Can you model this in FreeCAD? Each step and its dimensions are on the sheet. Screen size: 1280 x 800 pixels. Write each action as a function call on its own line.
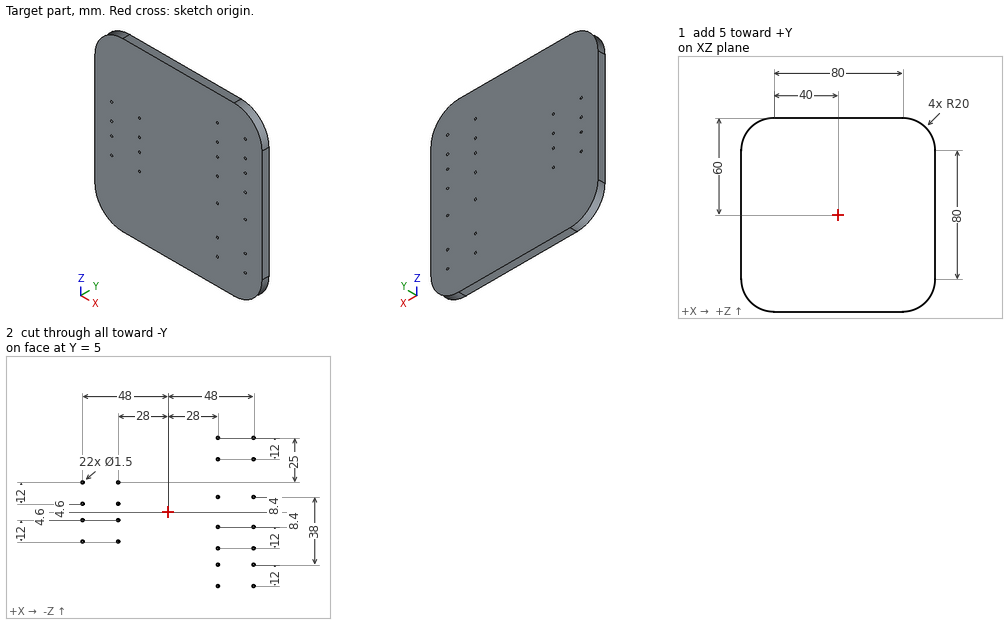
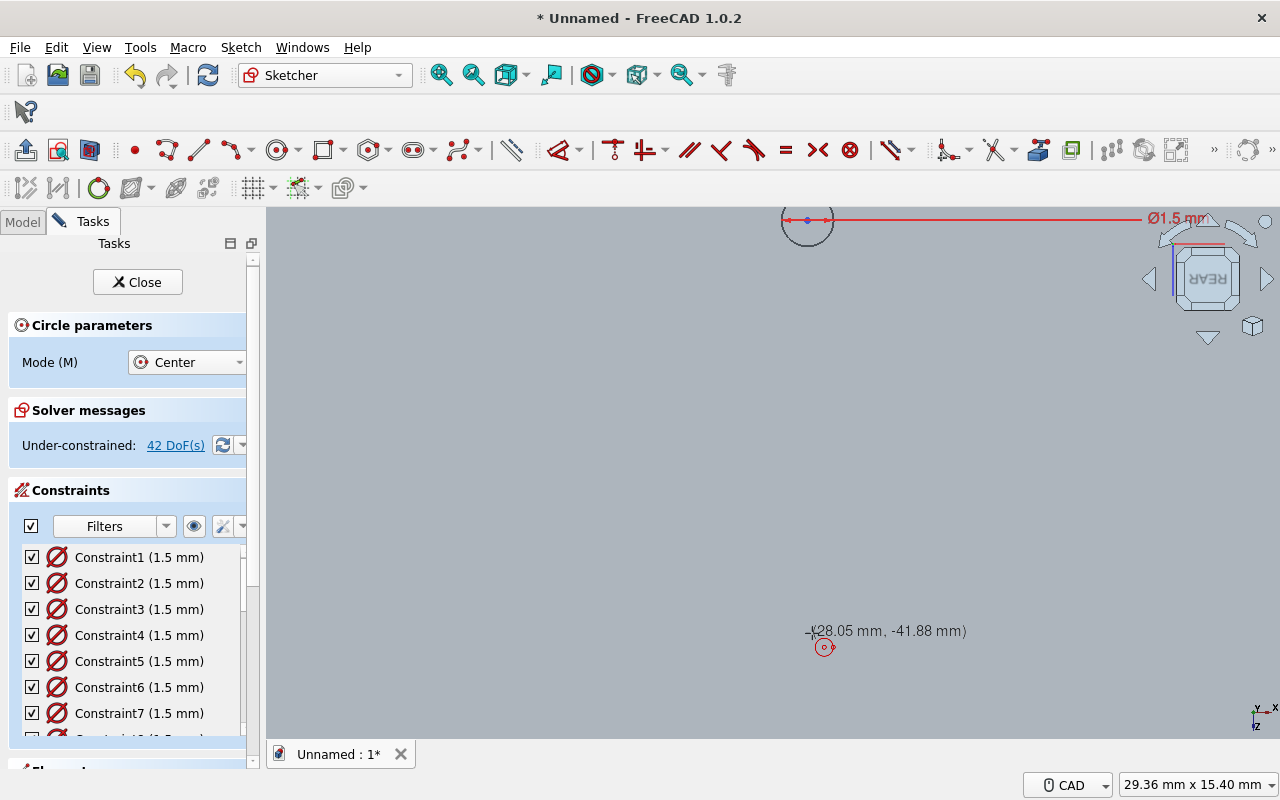
scroll(812, 633, down, 11)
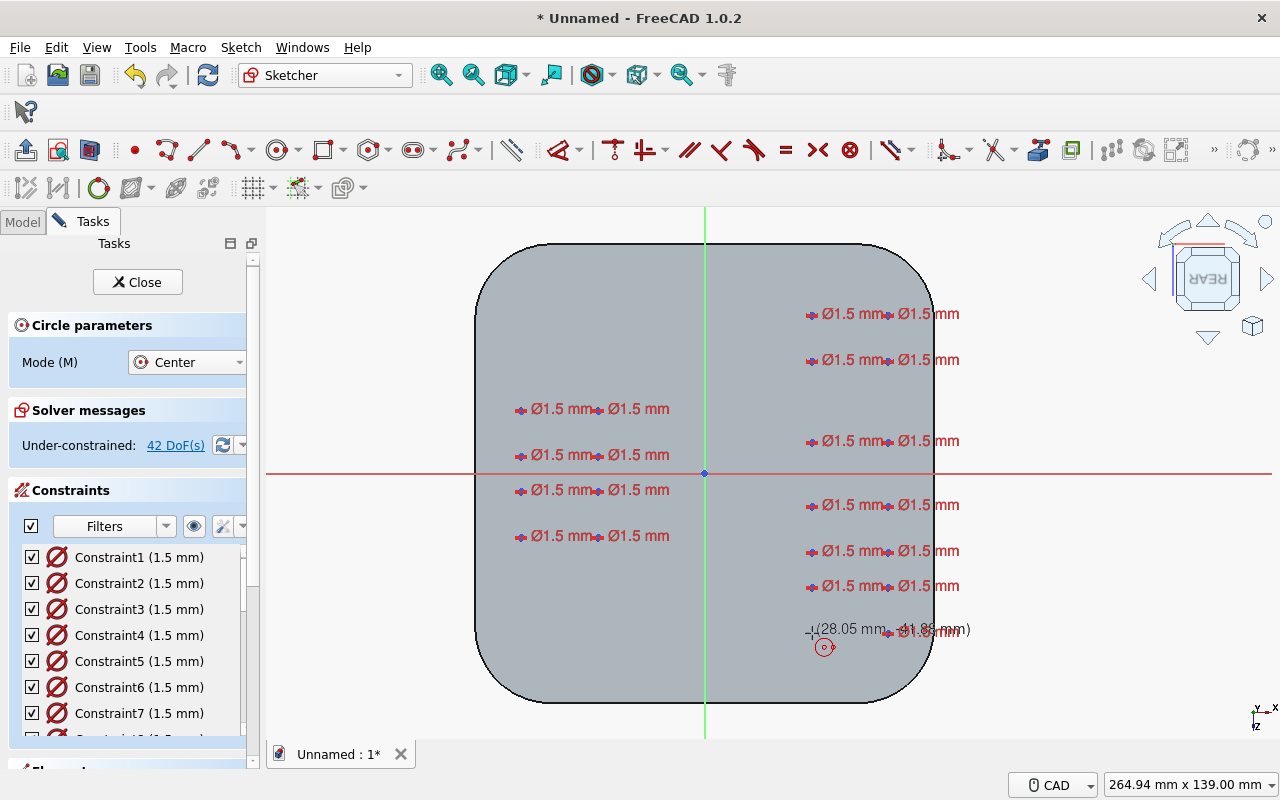
click(812, 633)
move(814, 631)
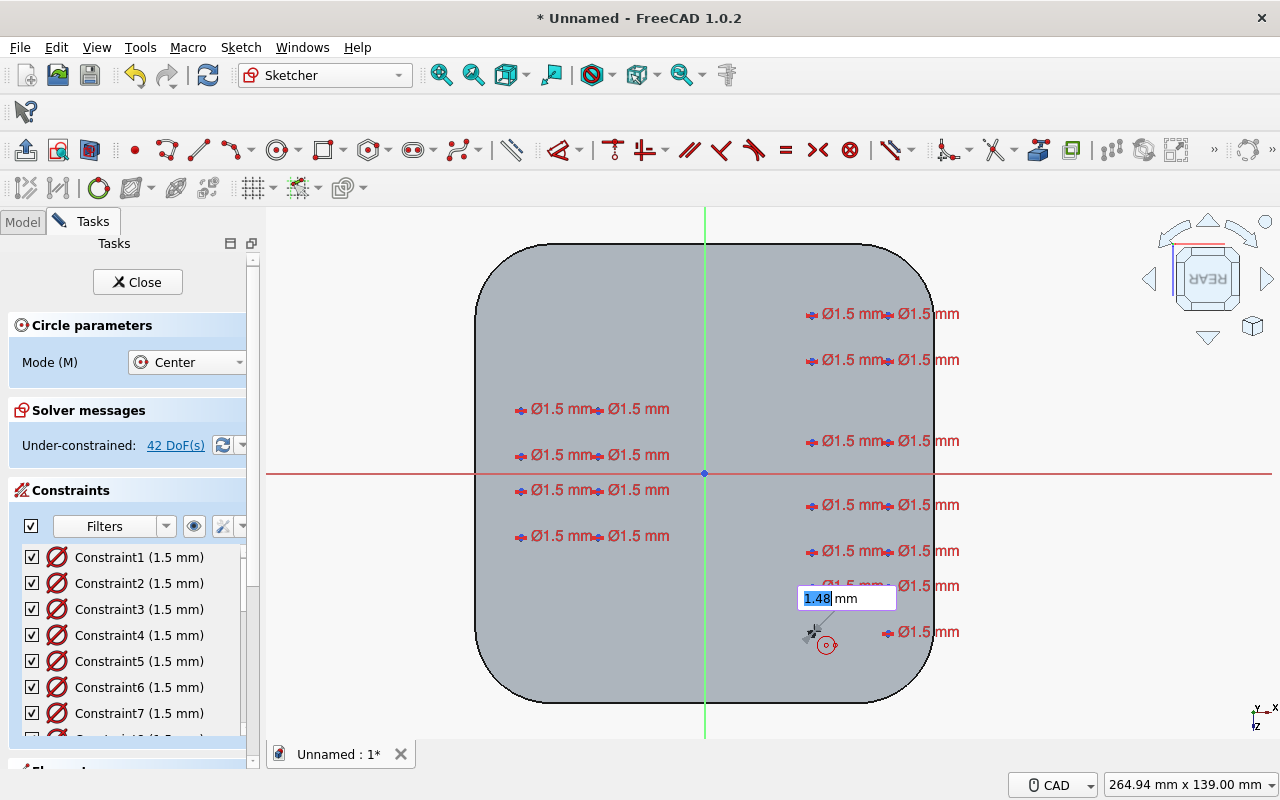
text(1.5)
key(Return)
key(Escape)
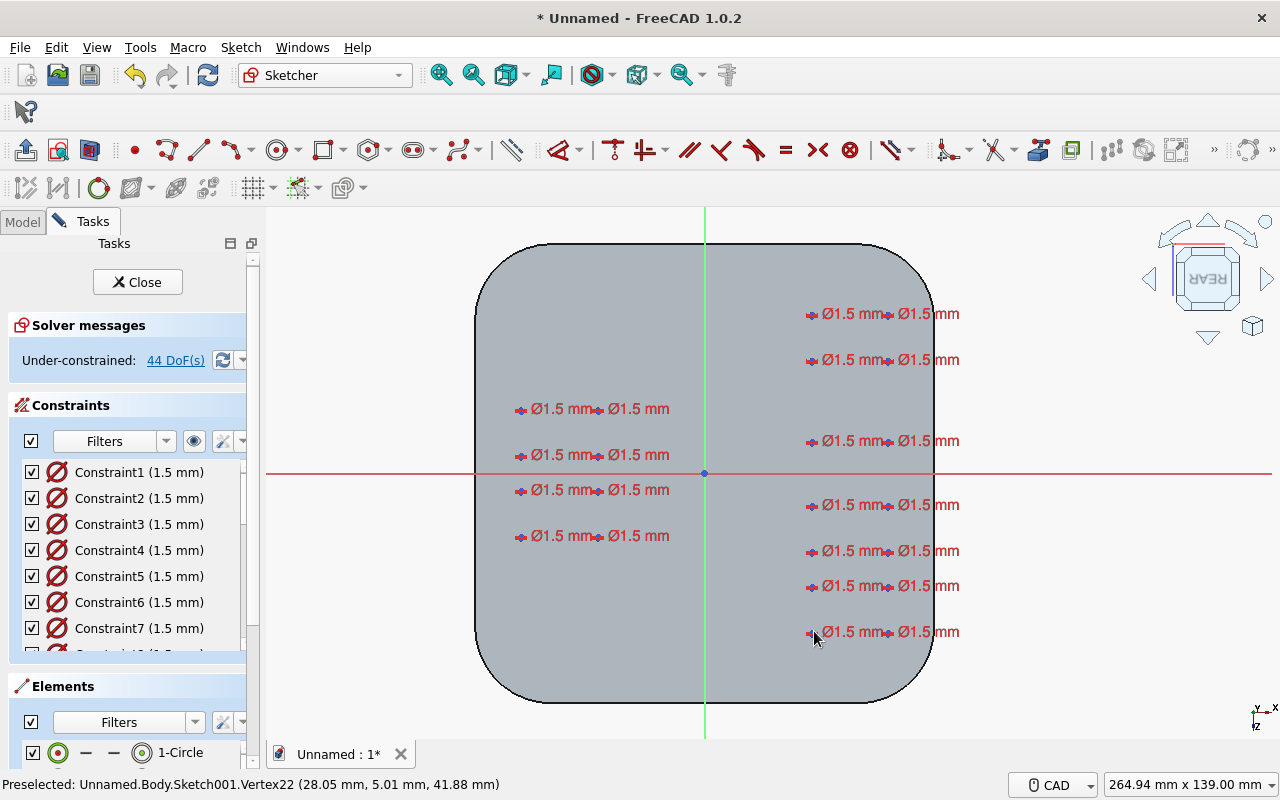
click(521, 411)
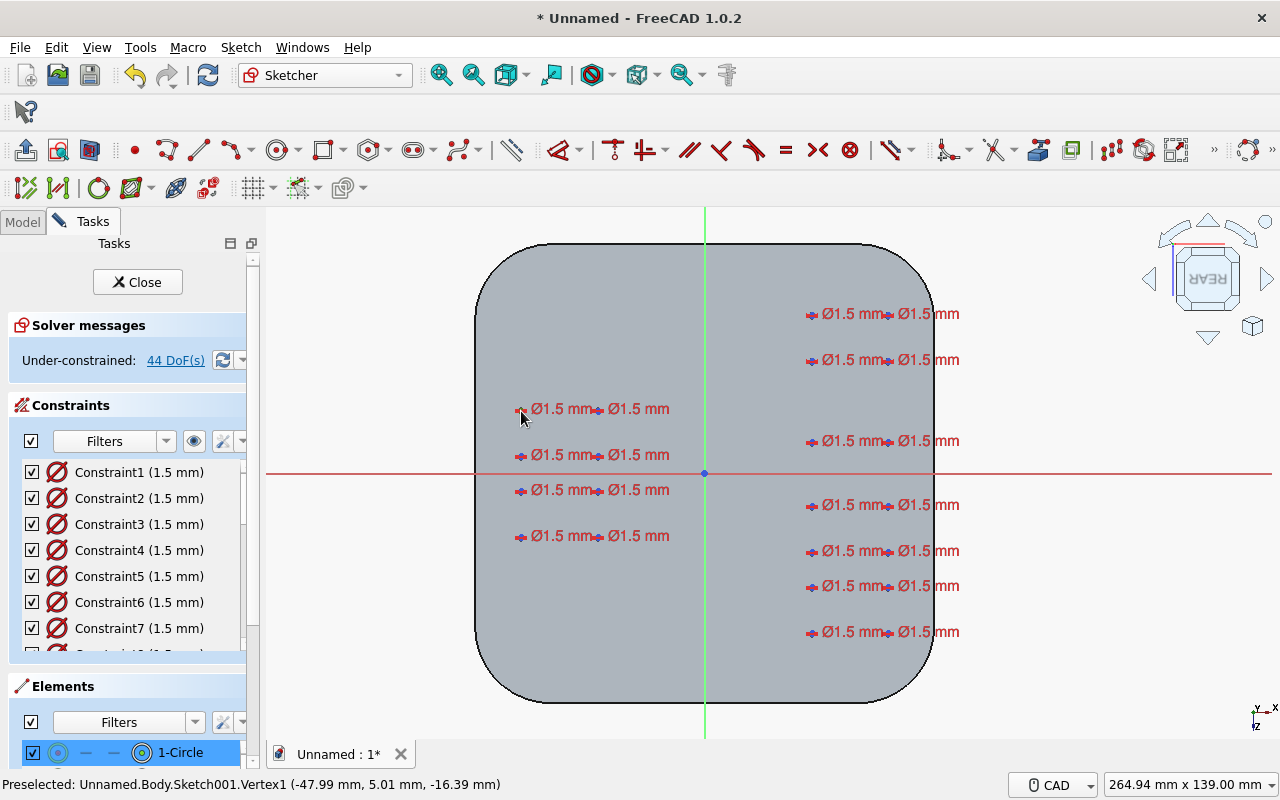
click(598, 411)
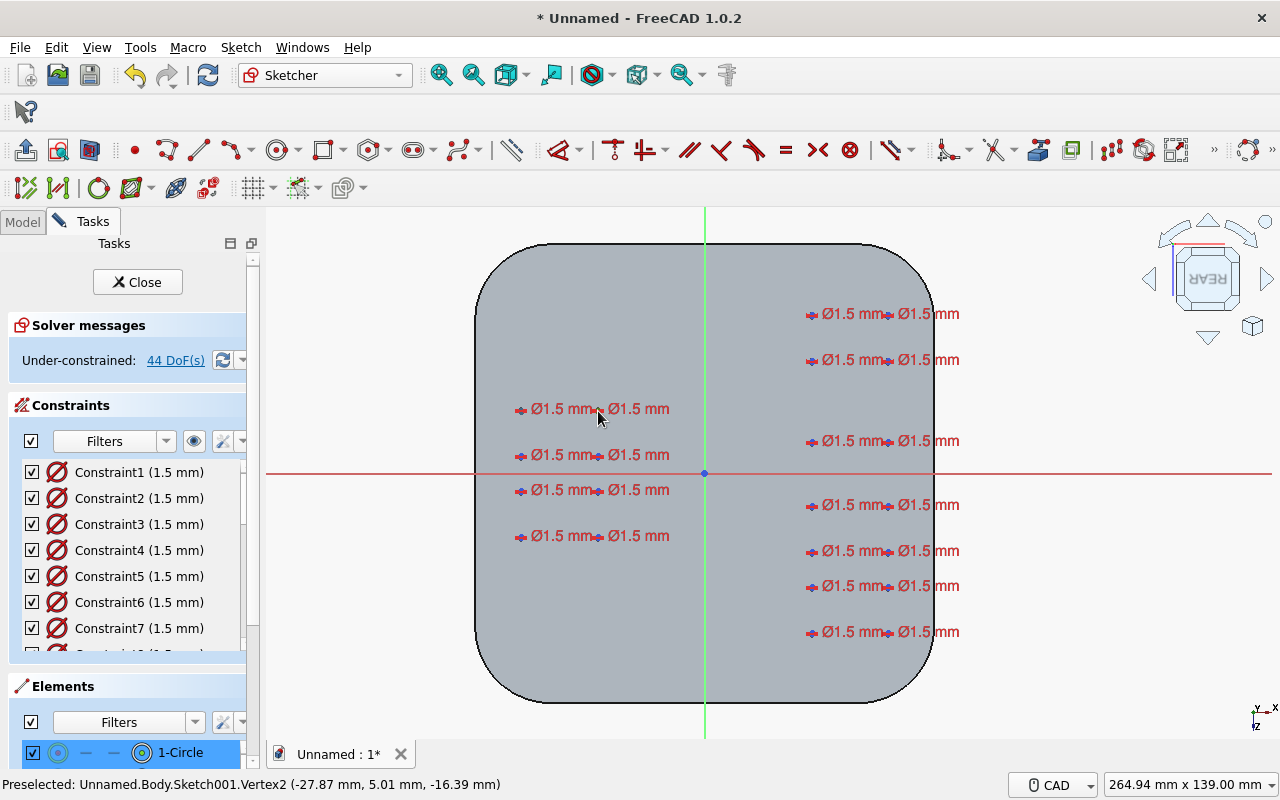
click(668, 150)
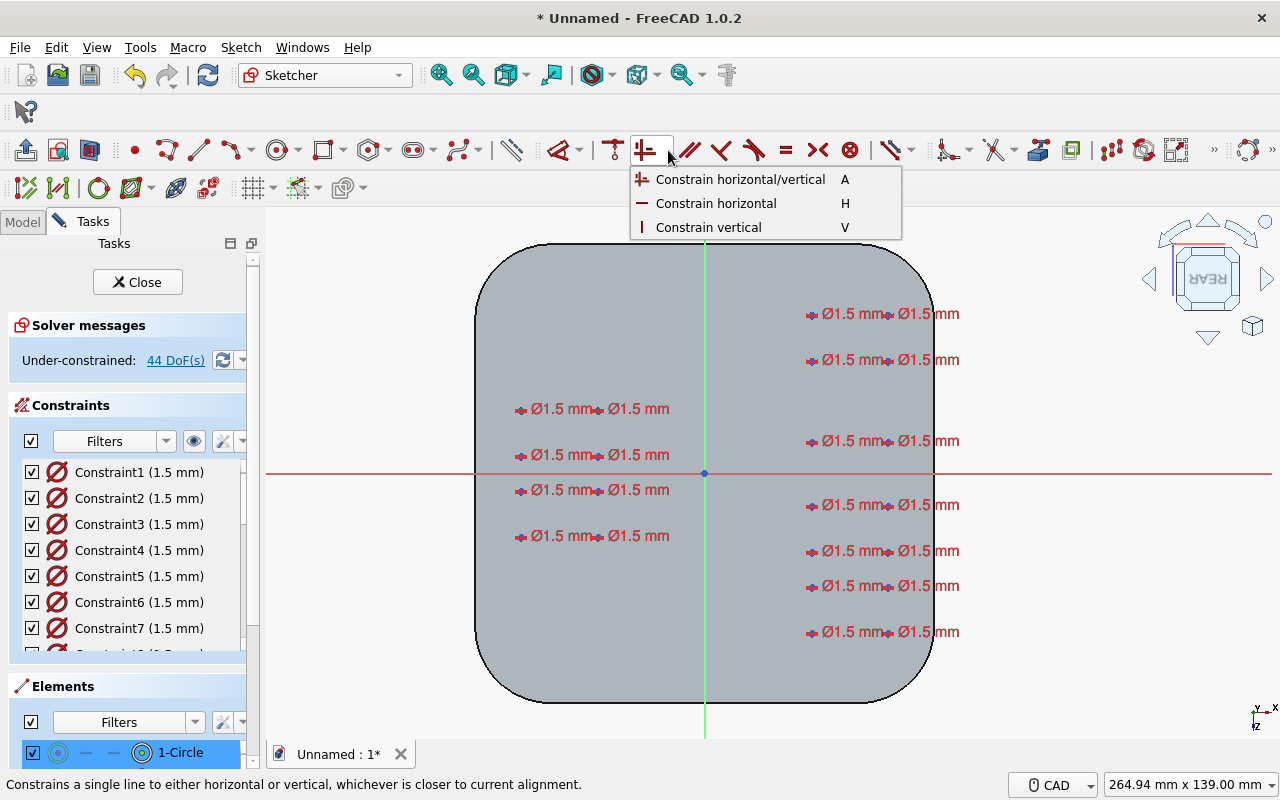
click(766, 203)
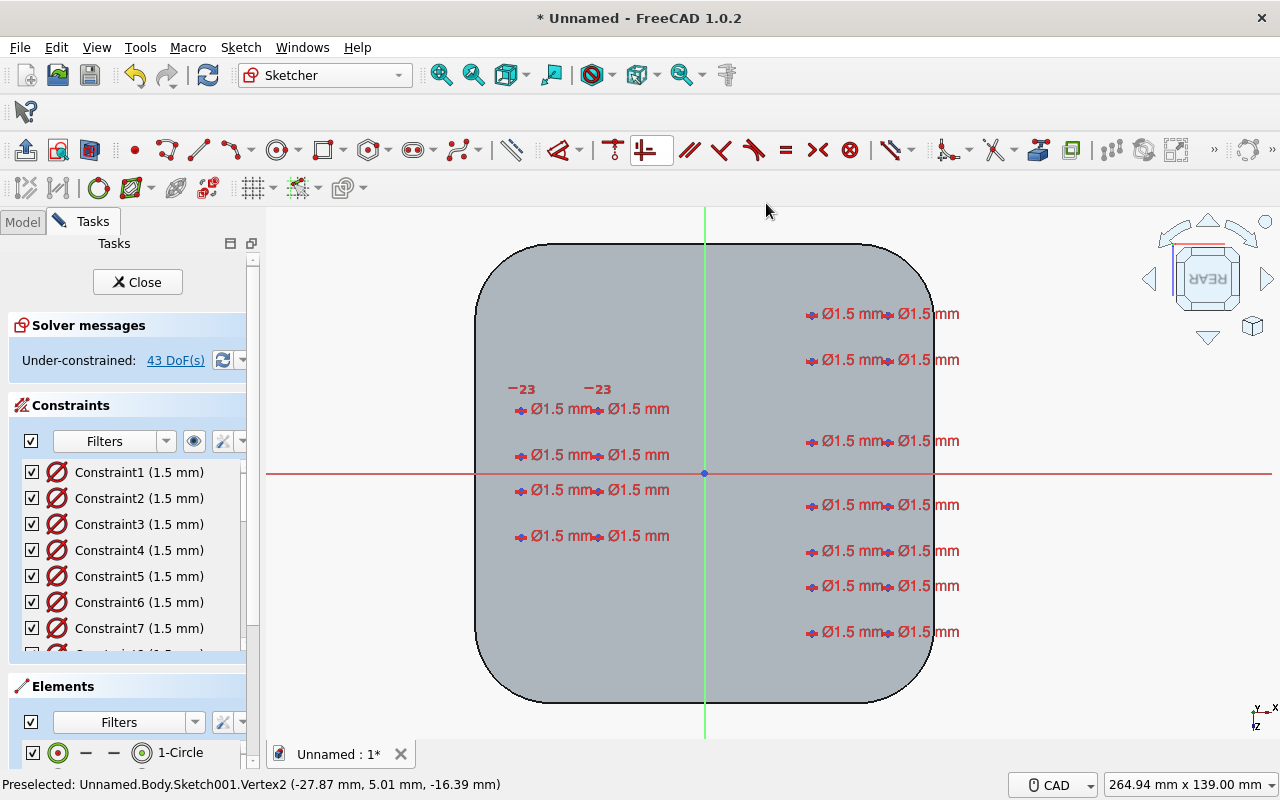
click(521, 411)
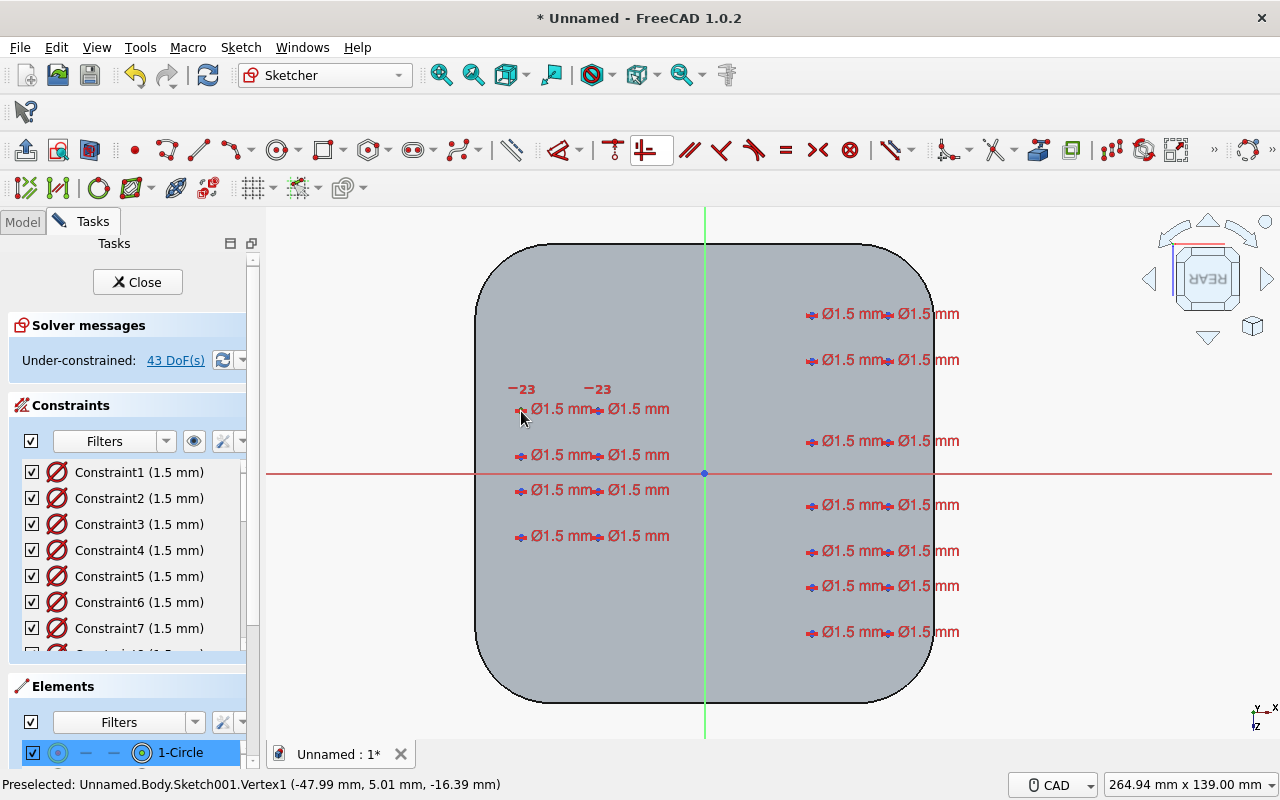
click(521, 457)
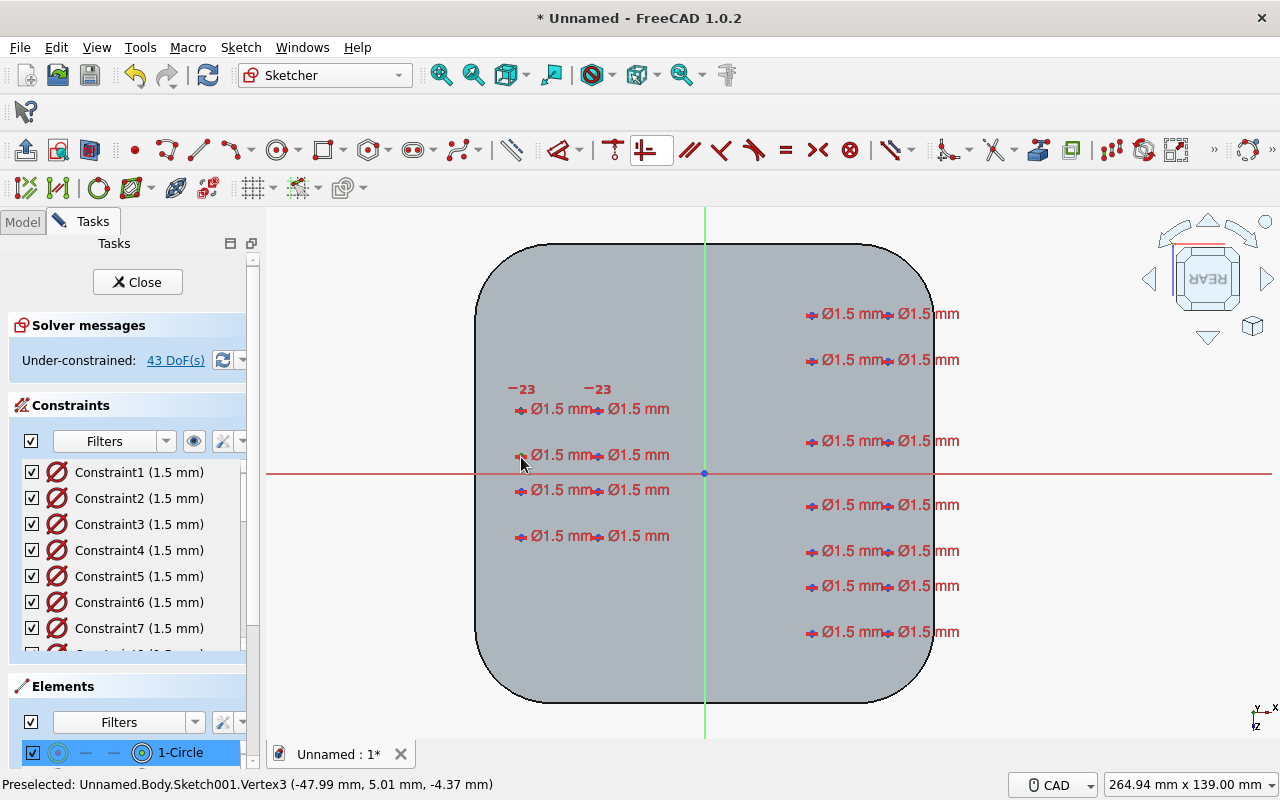
click(668, 150)